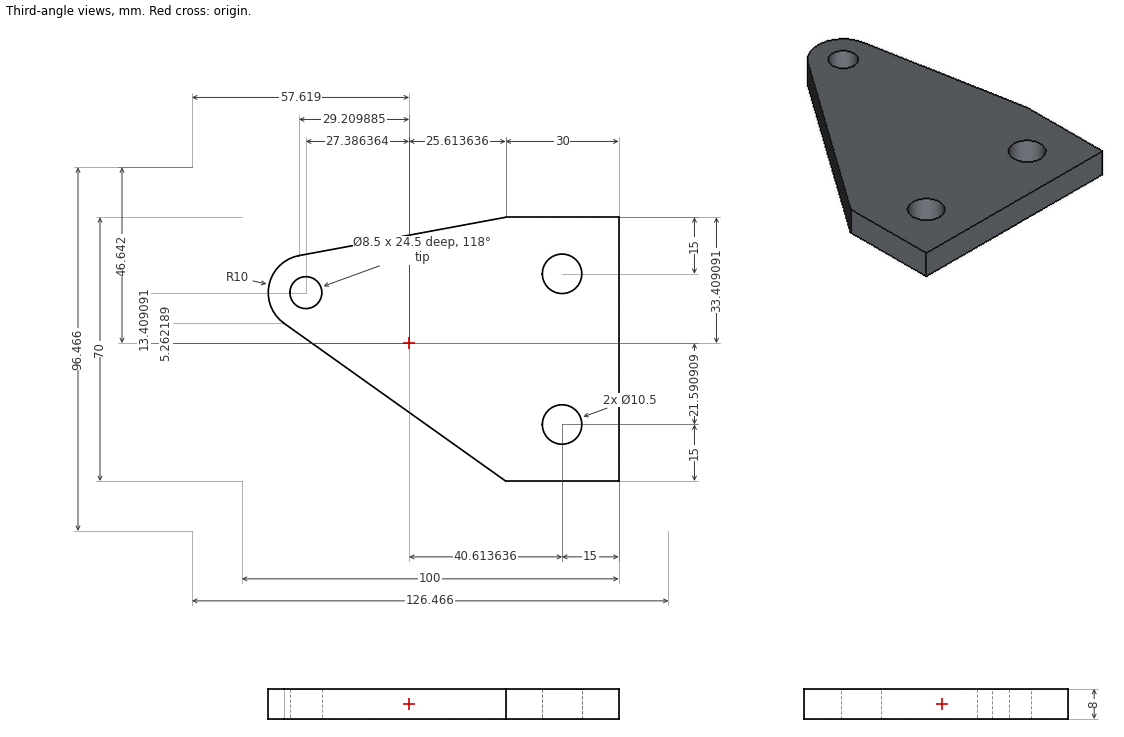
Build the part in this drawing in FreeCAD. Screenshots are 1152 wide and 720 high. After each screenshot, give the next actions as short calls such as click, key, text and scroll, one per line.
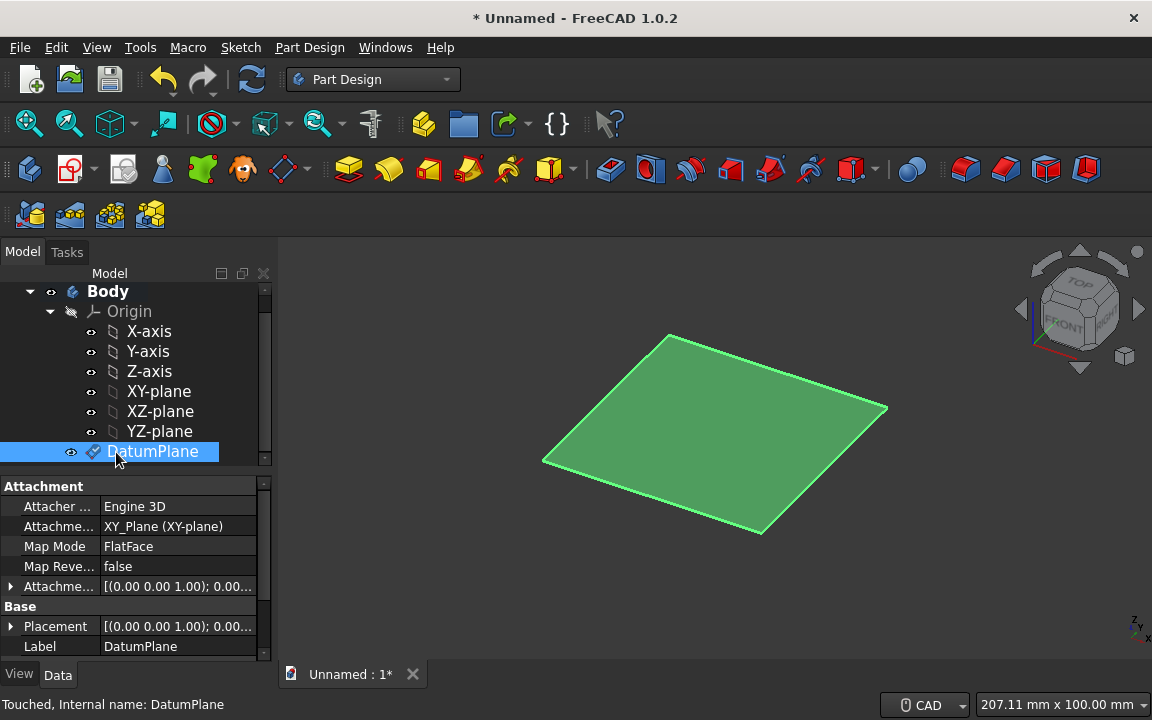
click(70, 170)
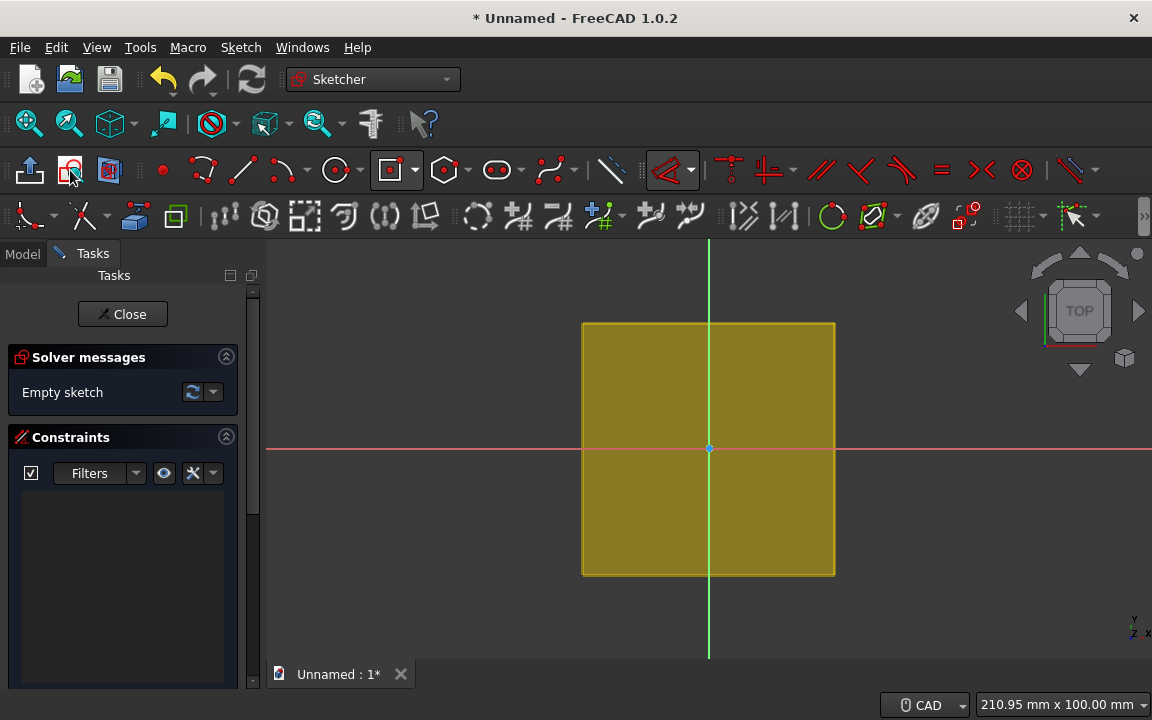
click(418, 170)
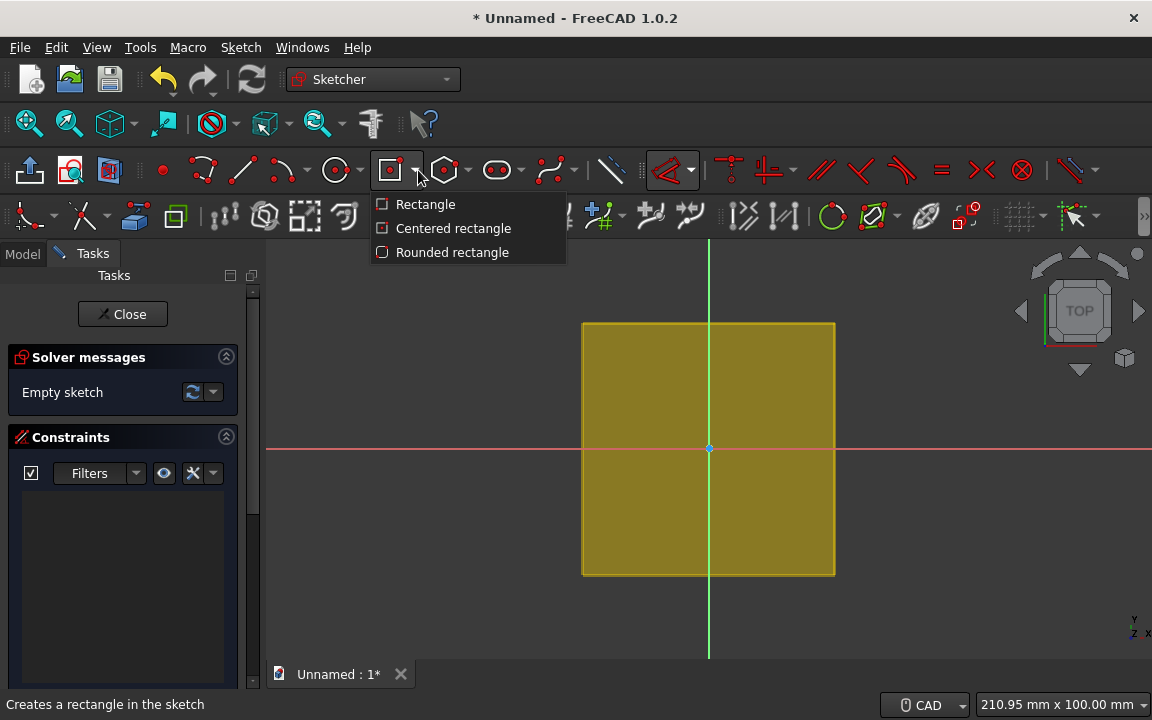
click(468, 204)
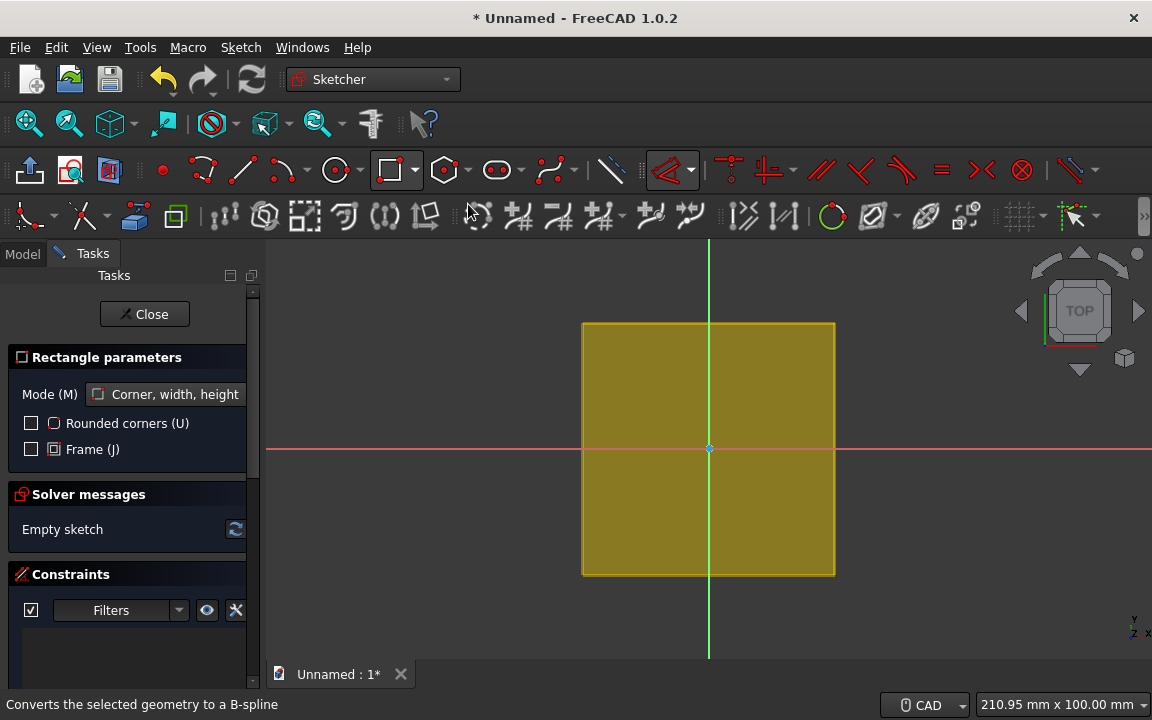
click(523, 309)
click(943, 603)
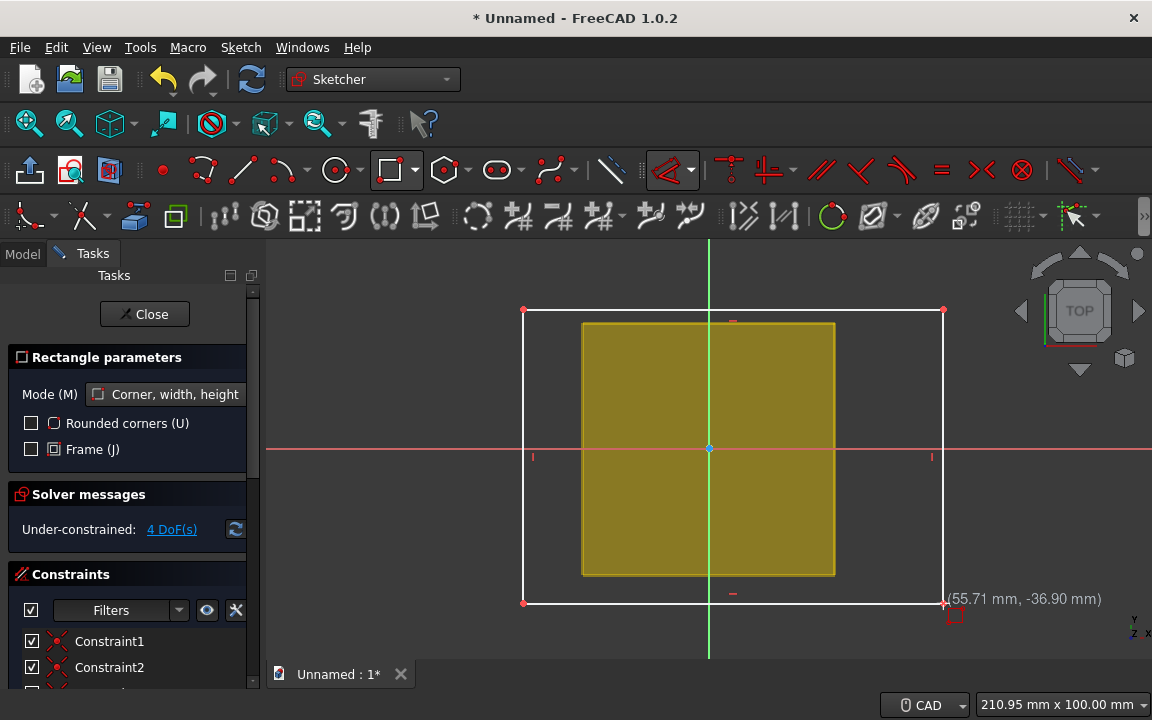
click(336, 170)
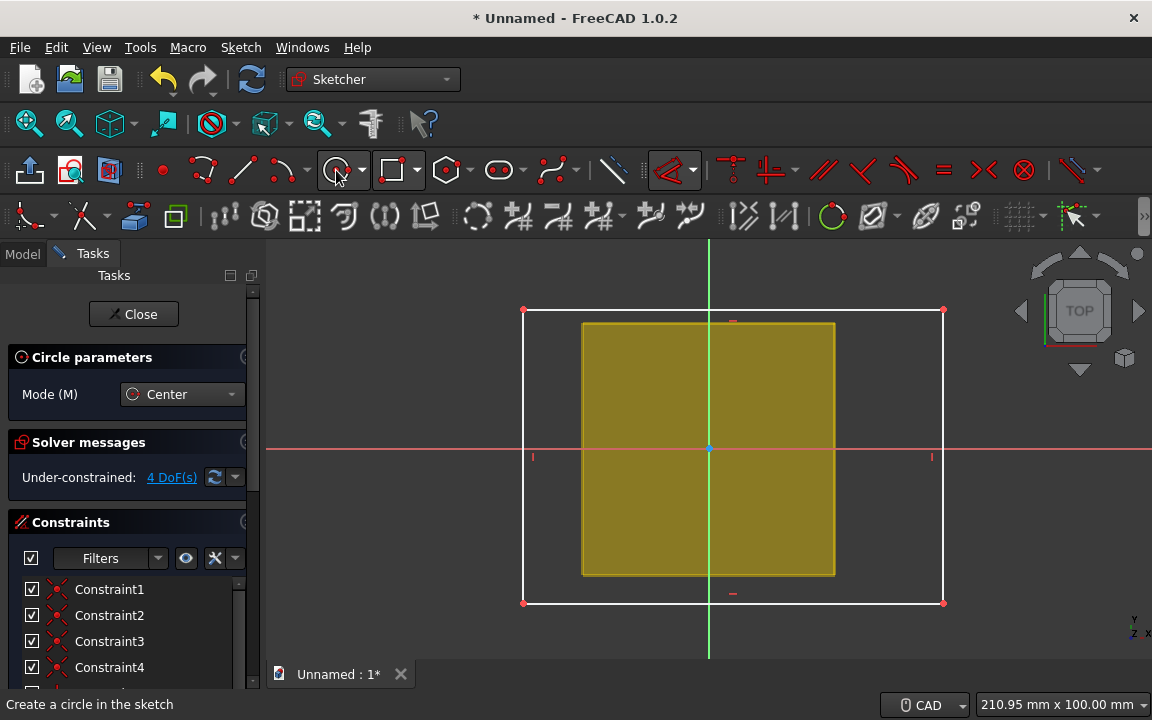
click(880, 540)
click(895, 524)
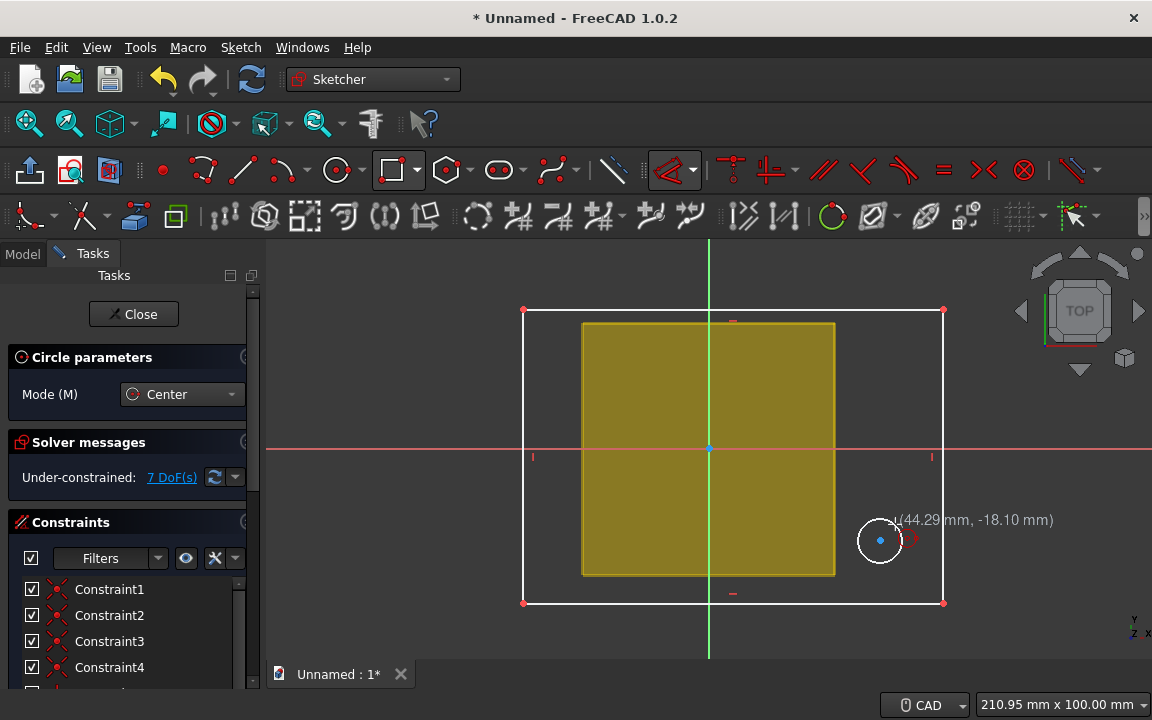
click(880, 372)
click(895, 356)
key(Escape)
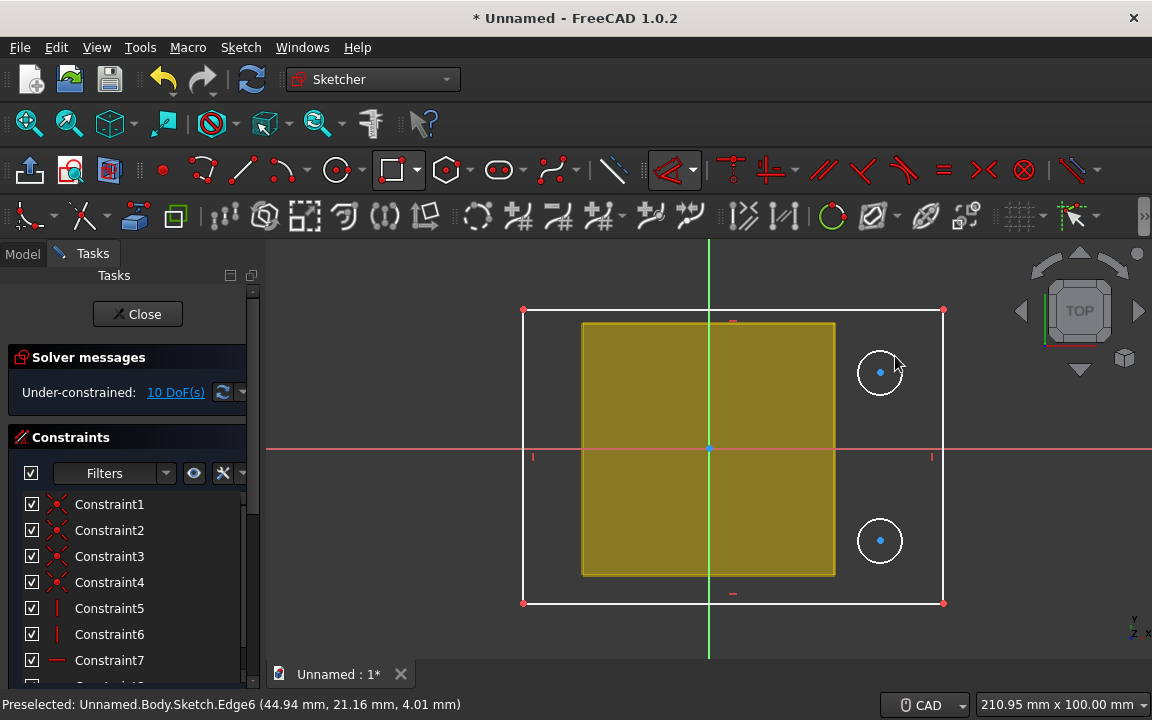
click(895, 525)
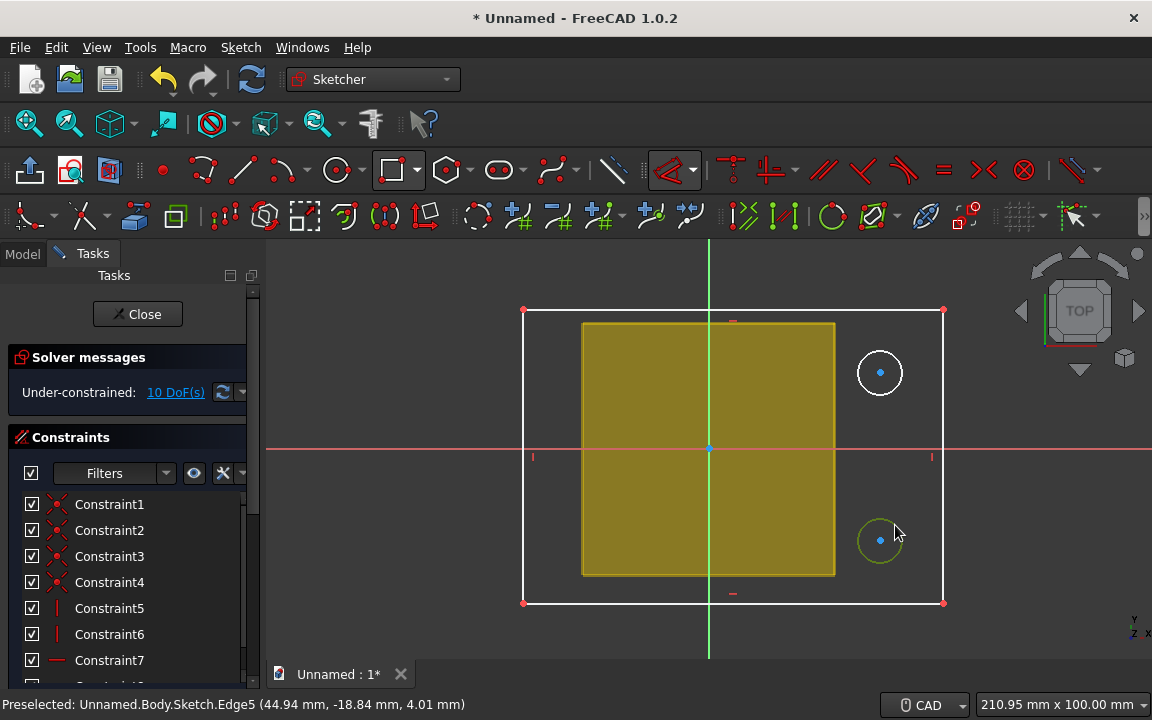
click(895, 357)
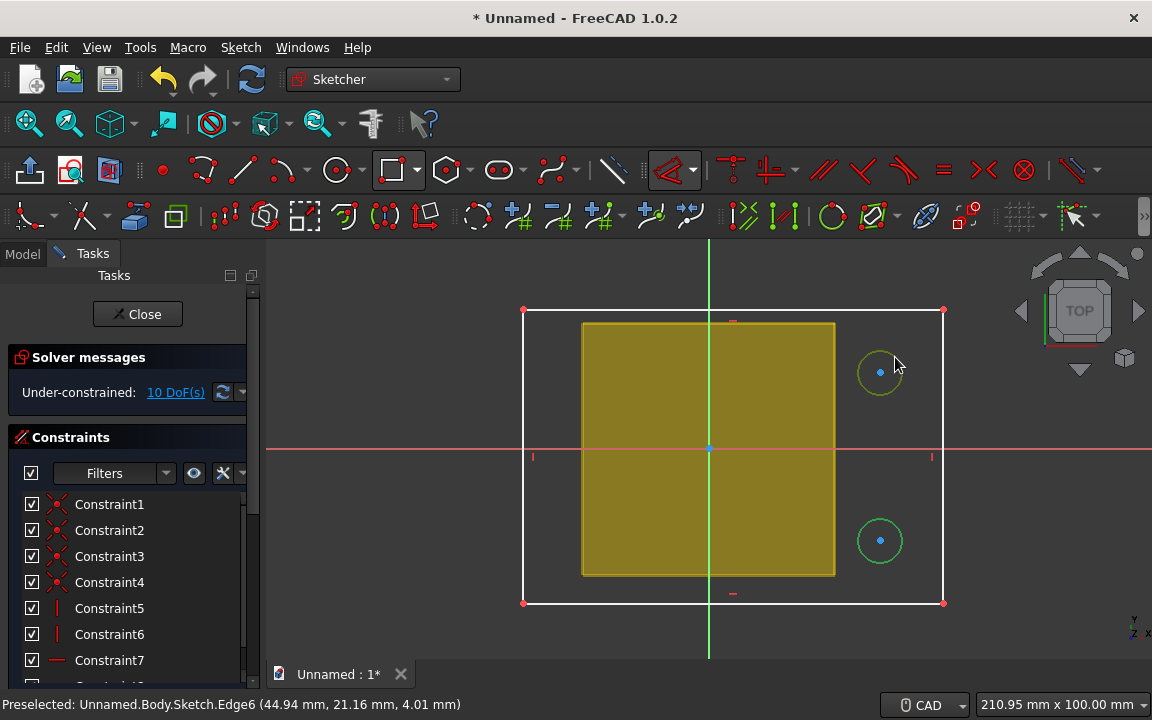
key(e)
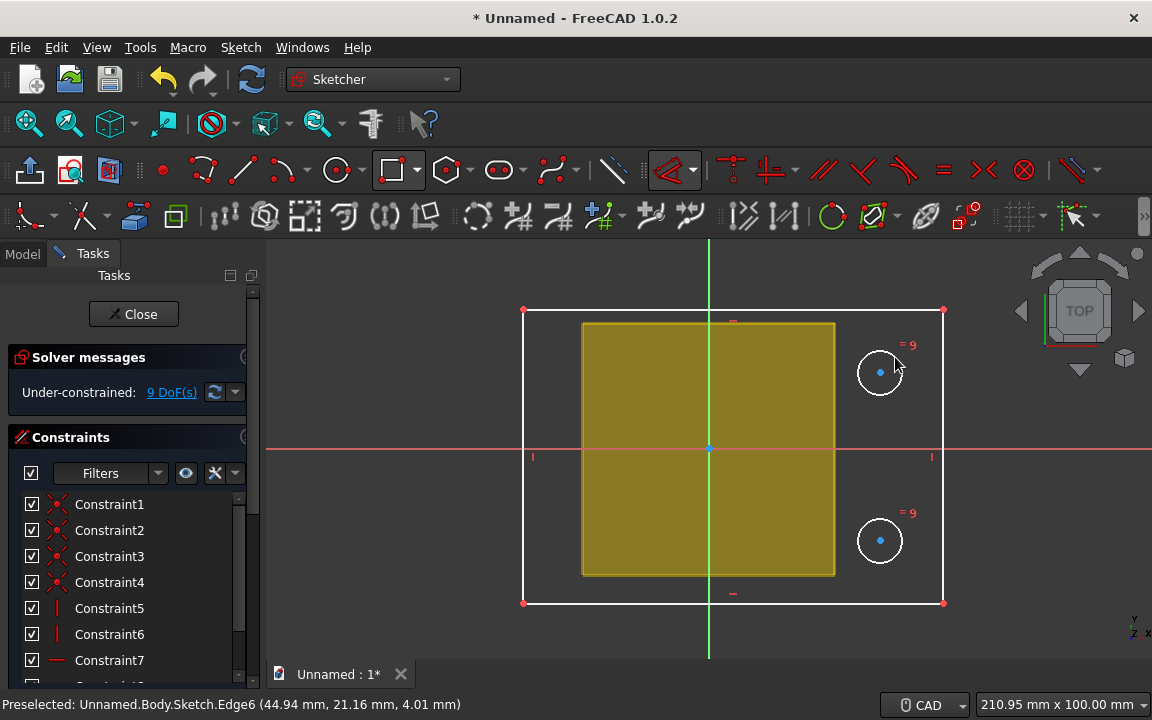
key(d)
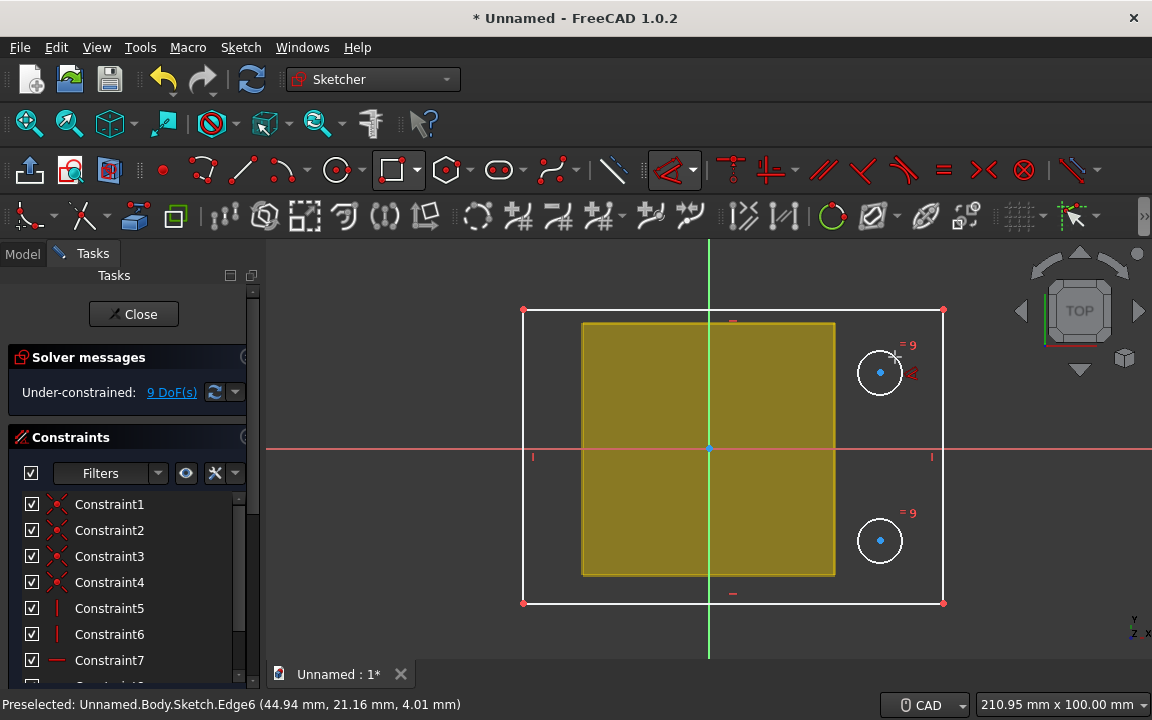
click(895, 525)
click(917, 502)